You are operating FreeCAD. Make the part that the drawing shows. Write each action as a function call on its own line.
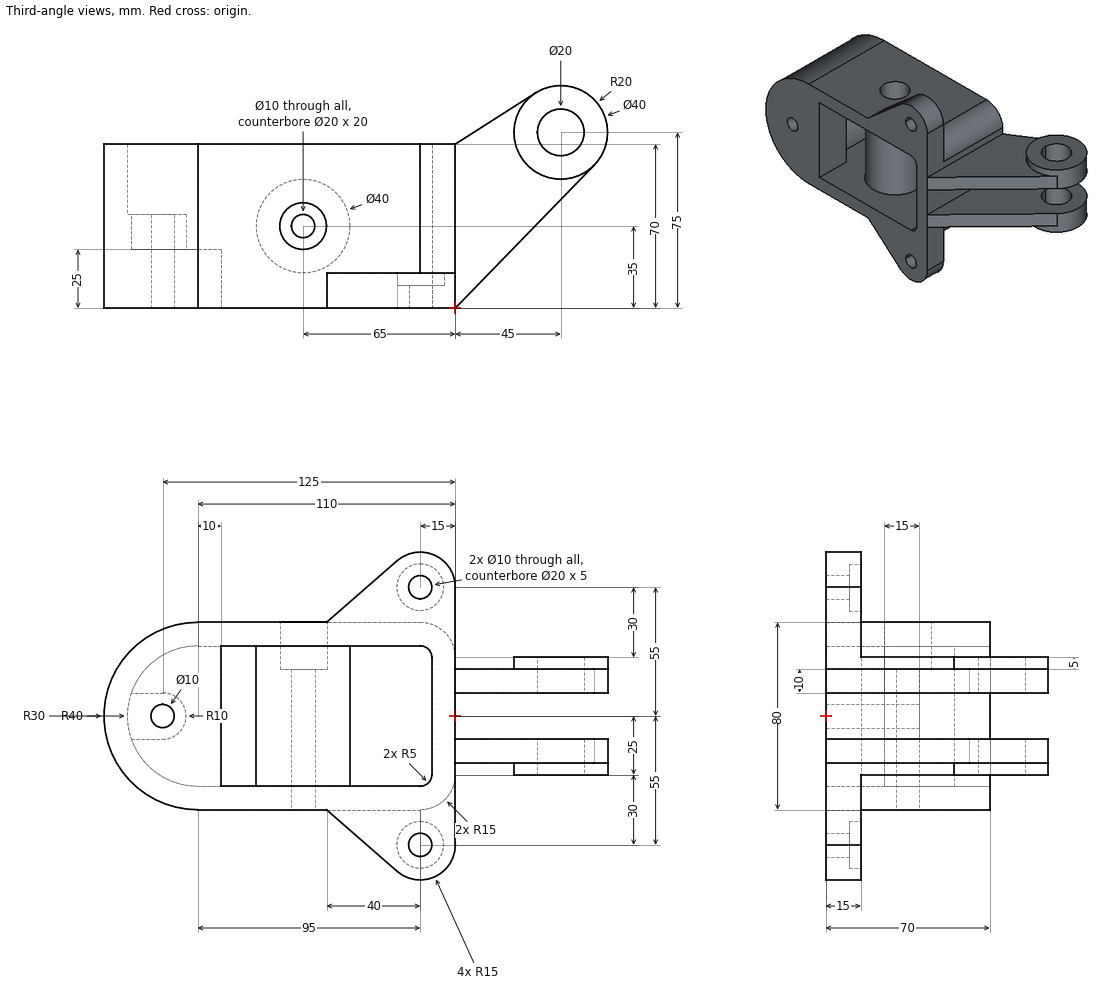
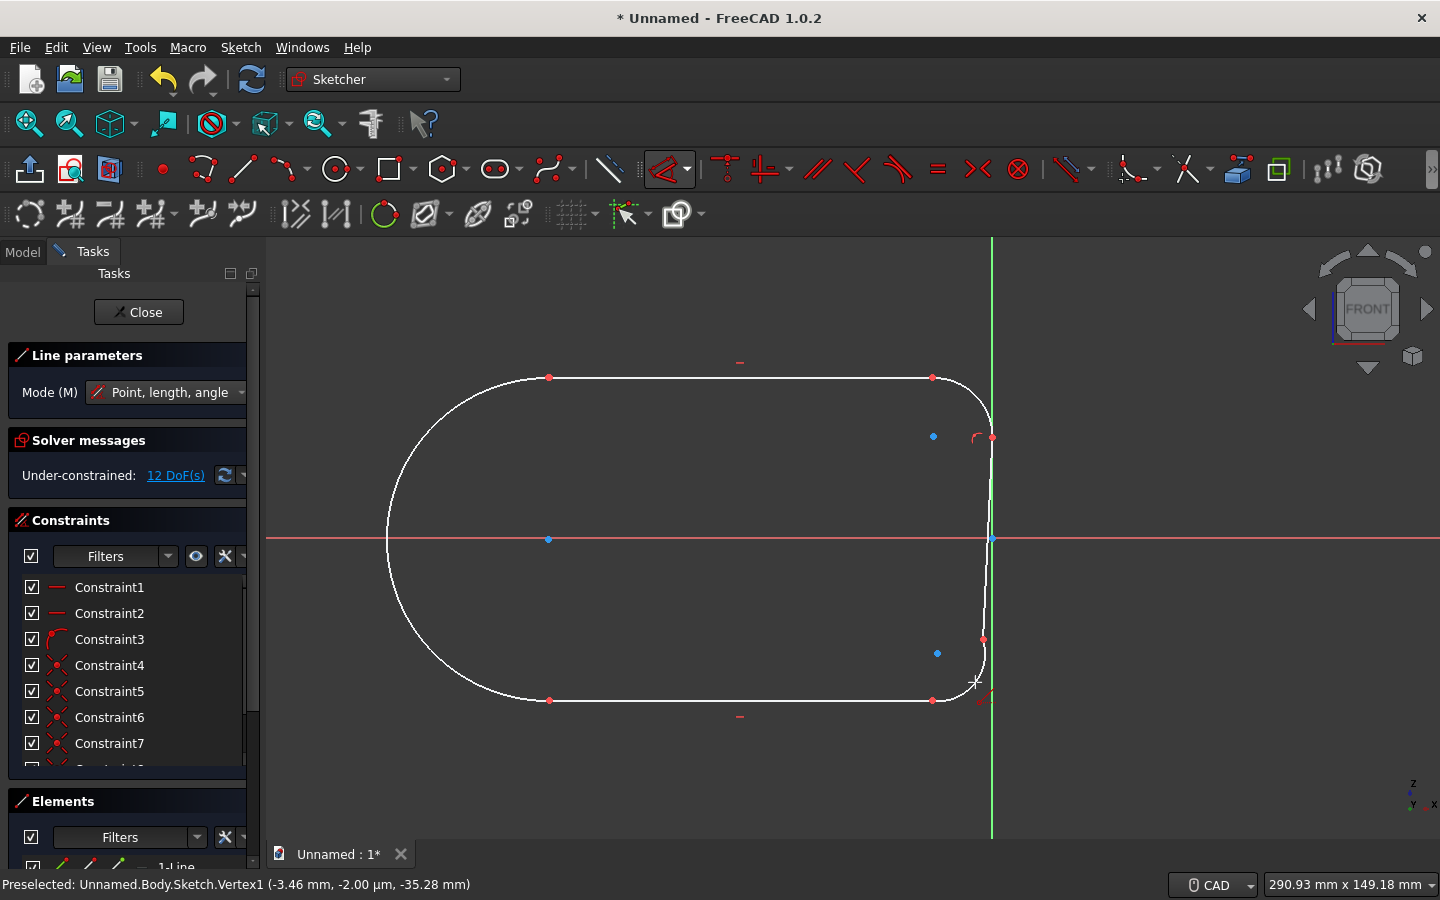
click(549, 659)
click(932, 659)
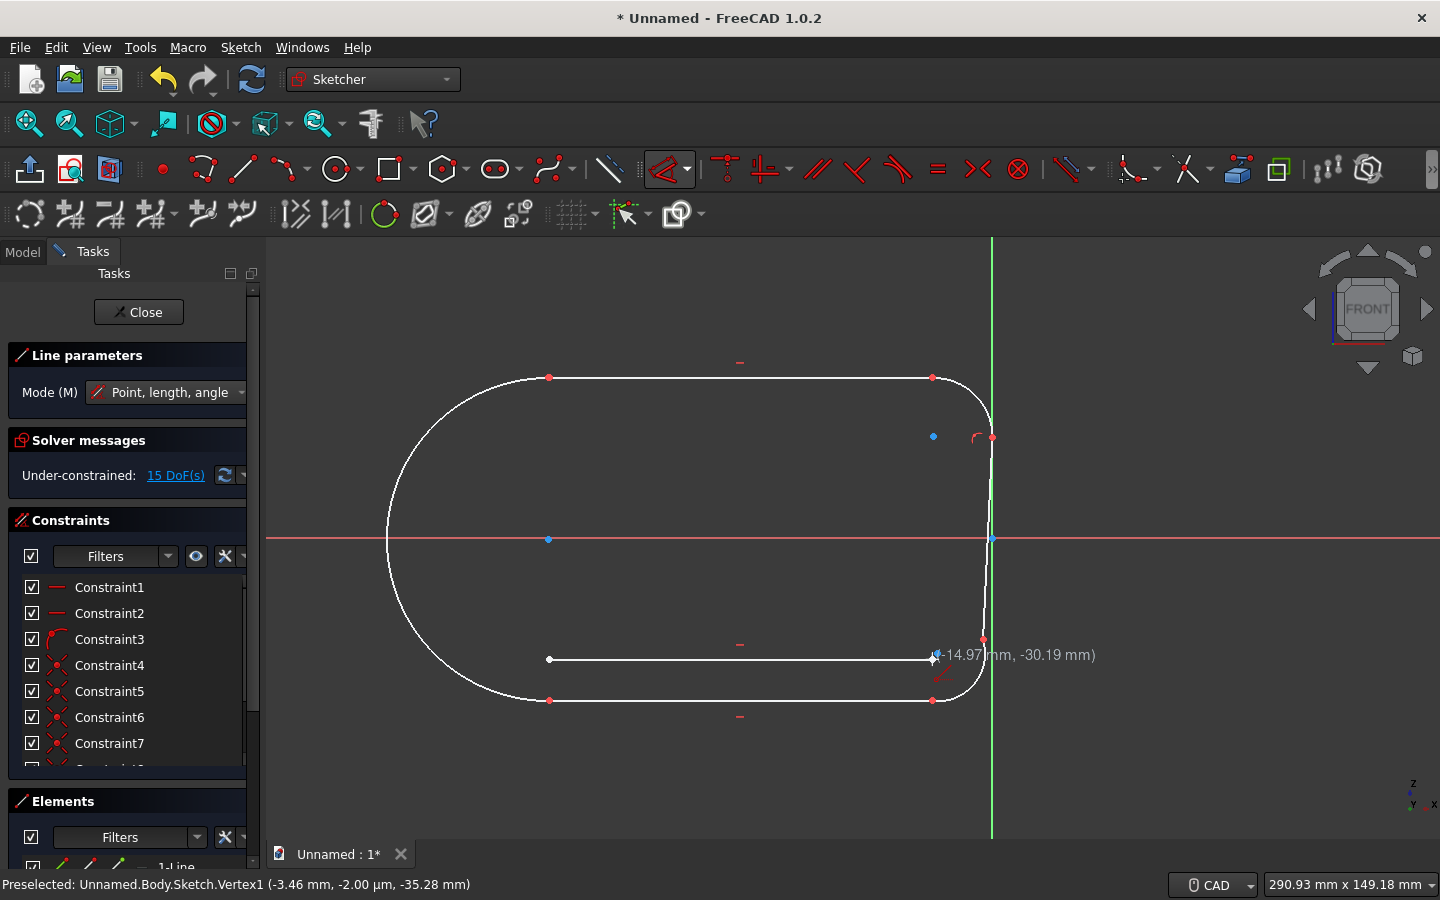
click(952, 639)
click(952, 437)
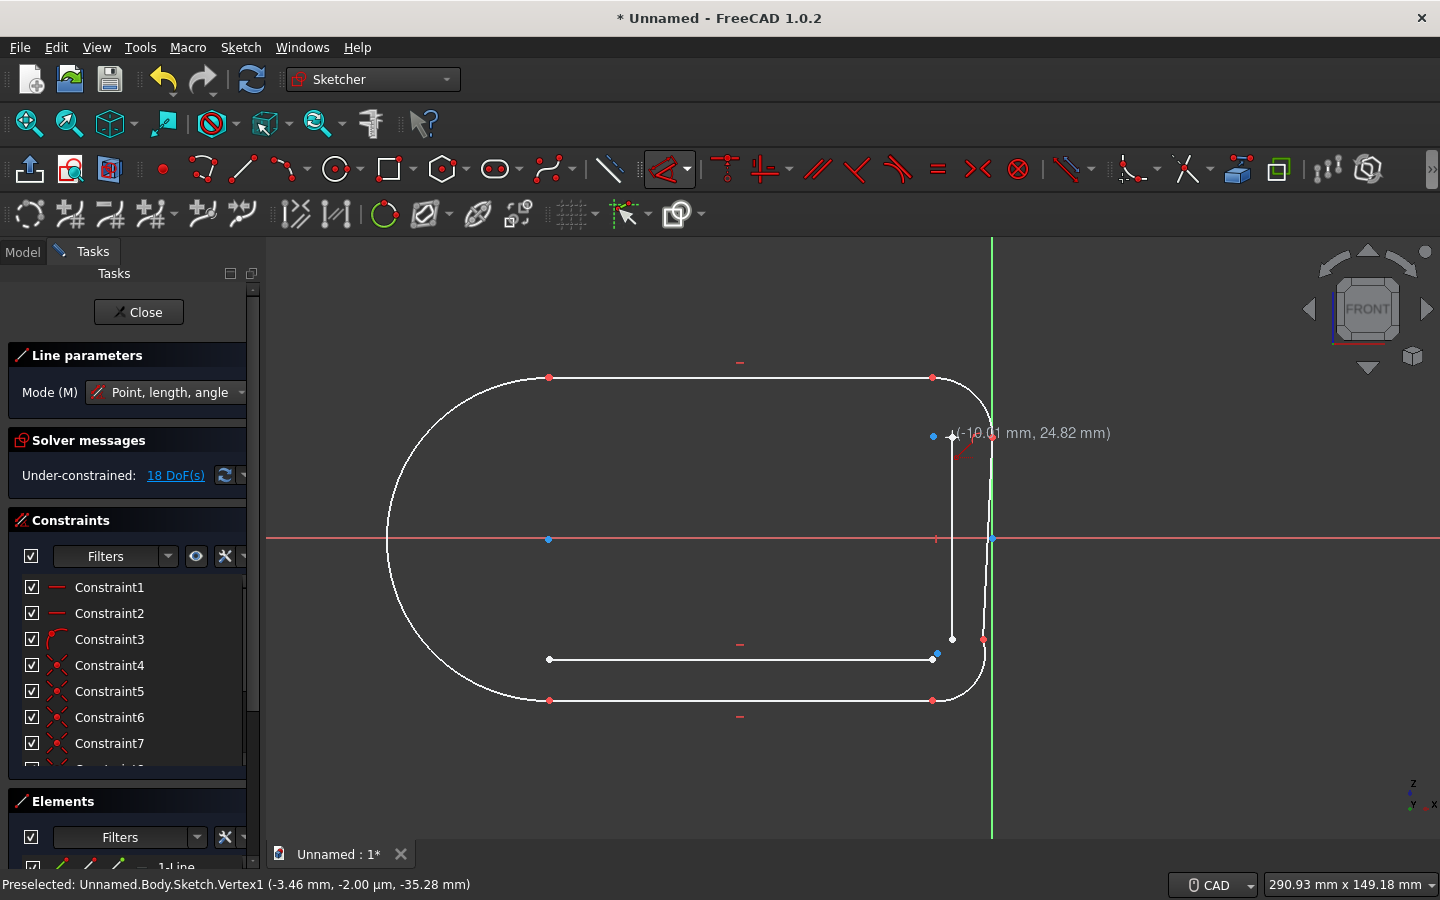
click(932, 417)
click(549, 417)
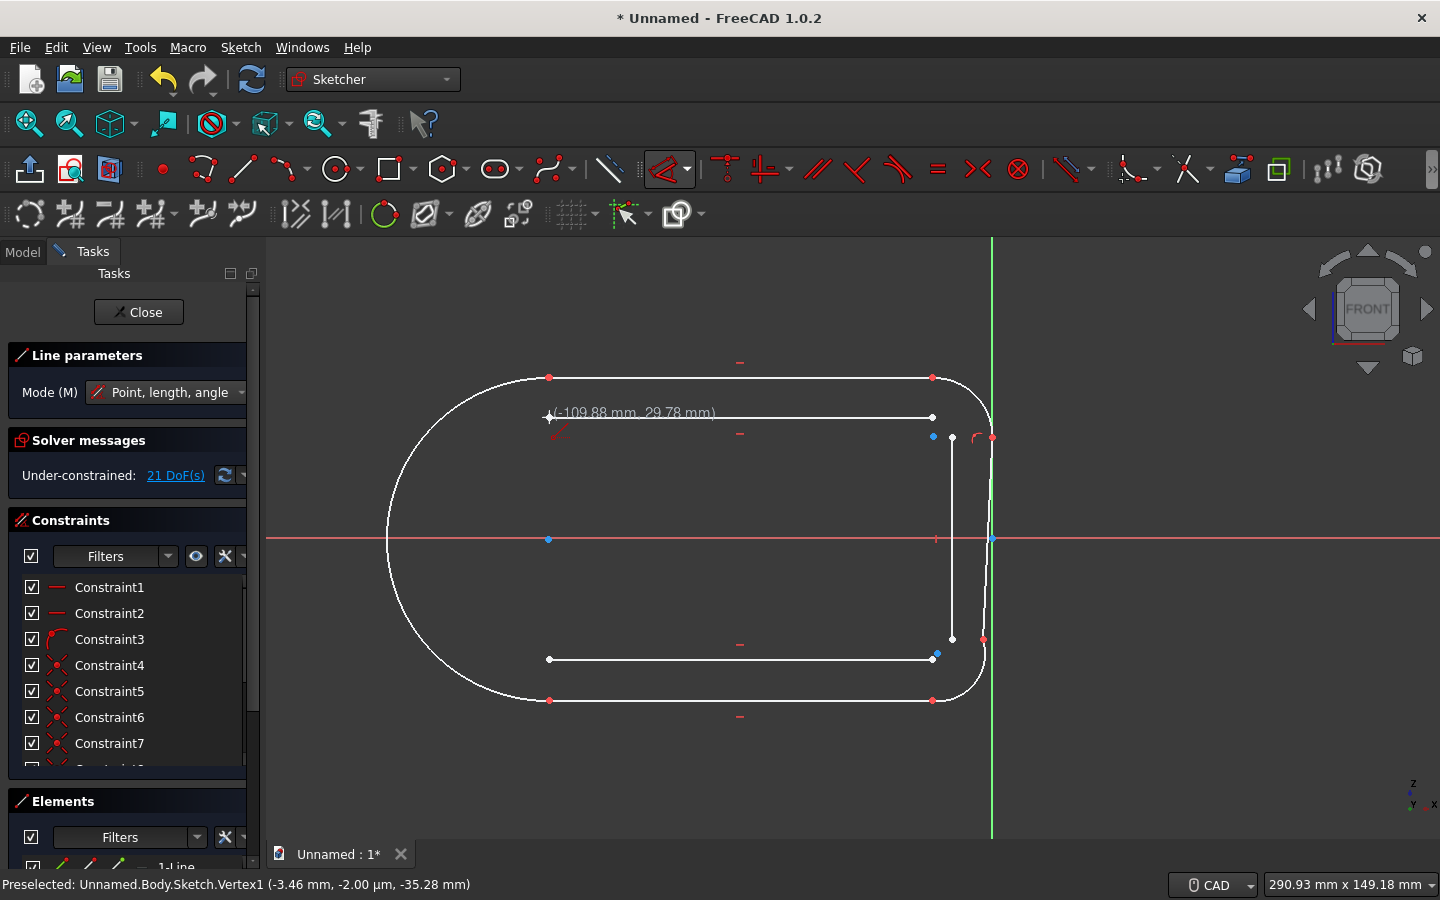
click(284, 170)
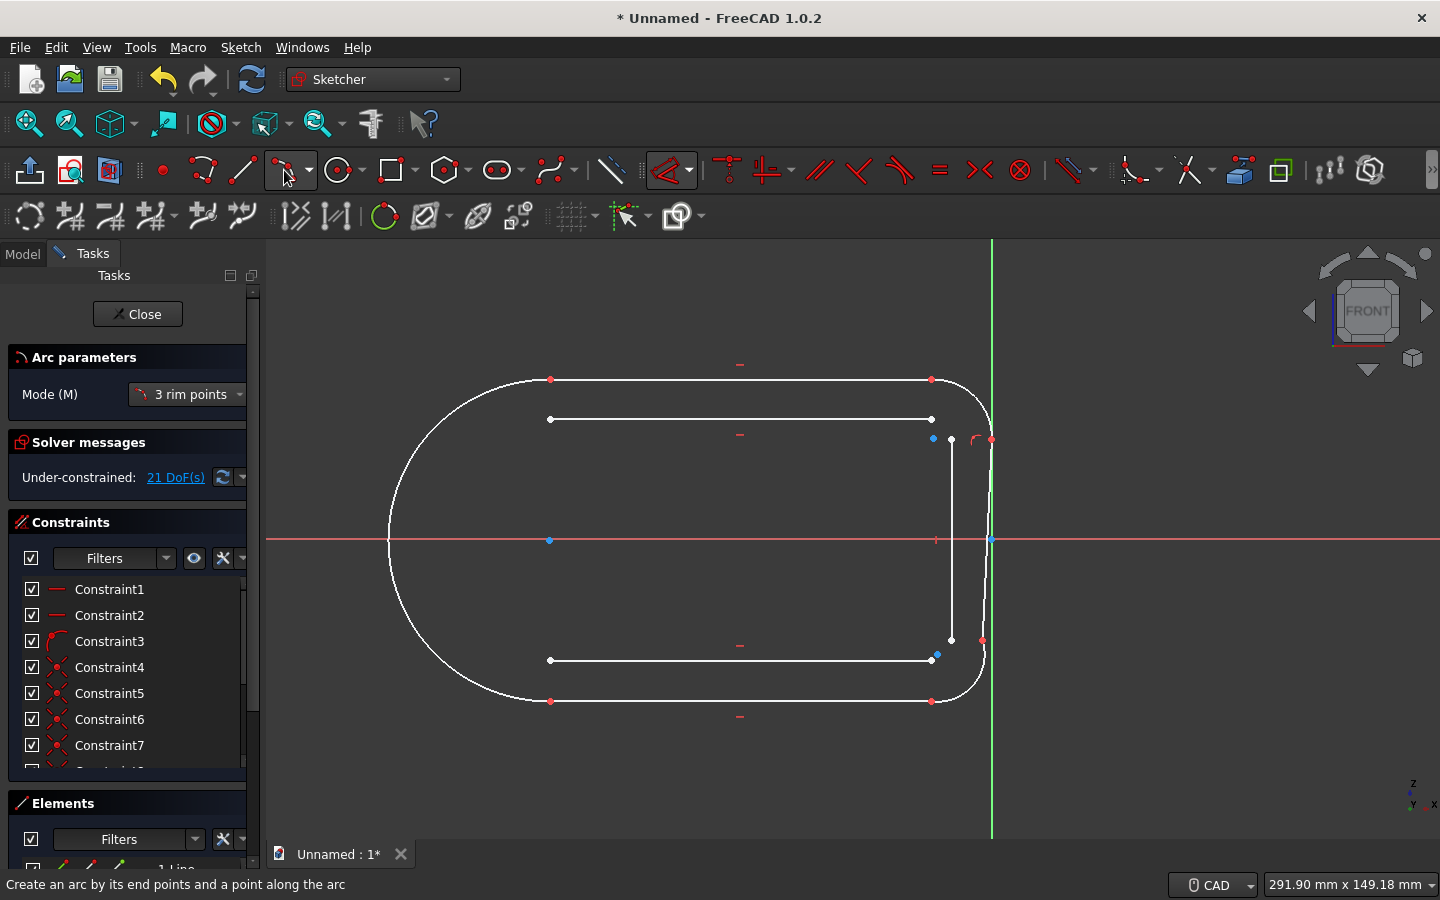
click(932, 661)
click(952, 641)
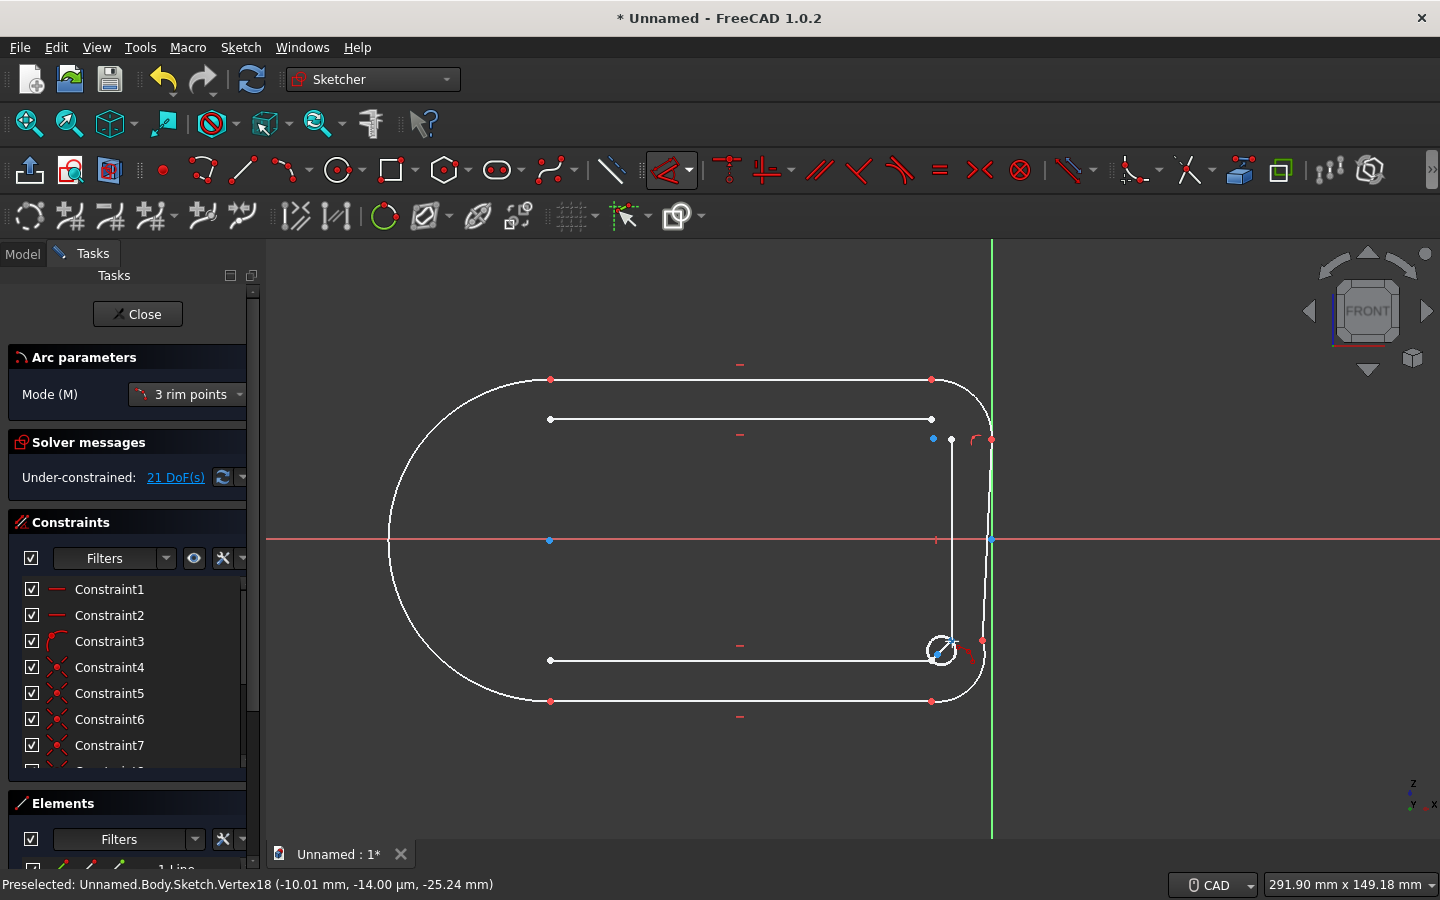
scroll(946, 654, up, 5)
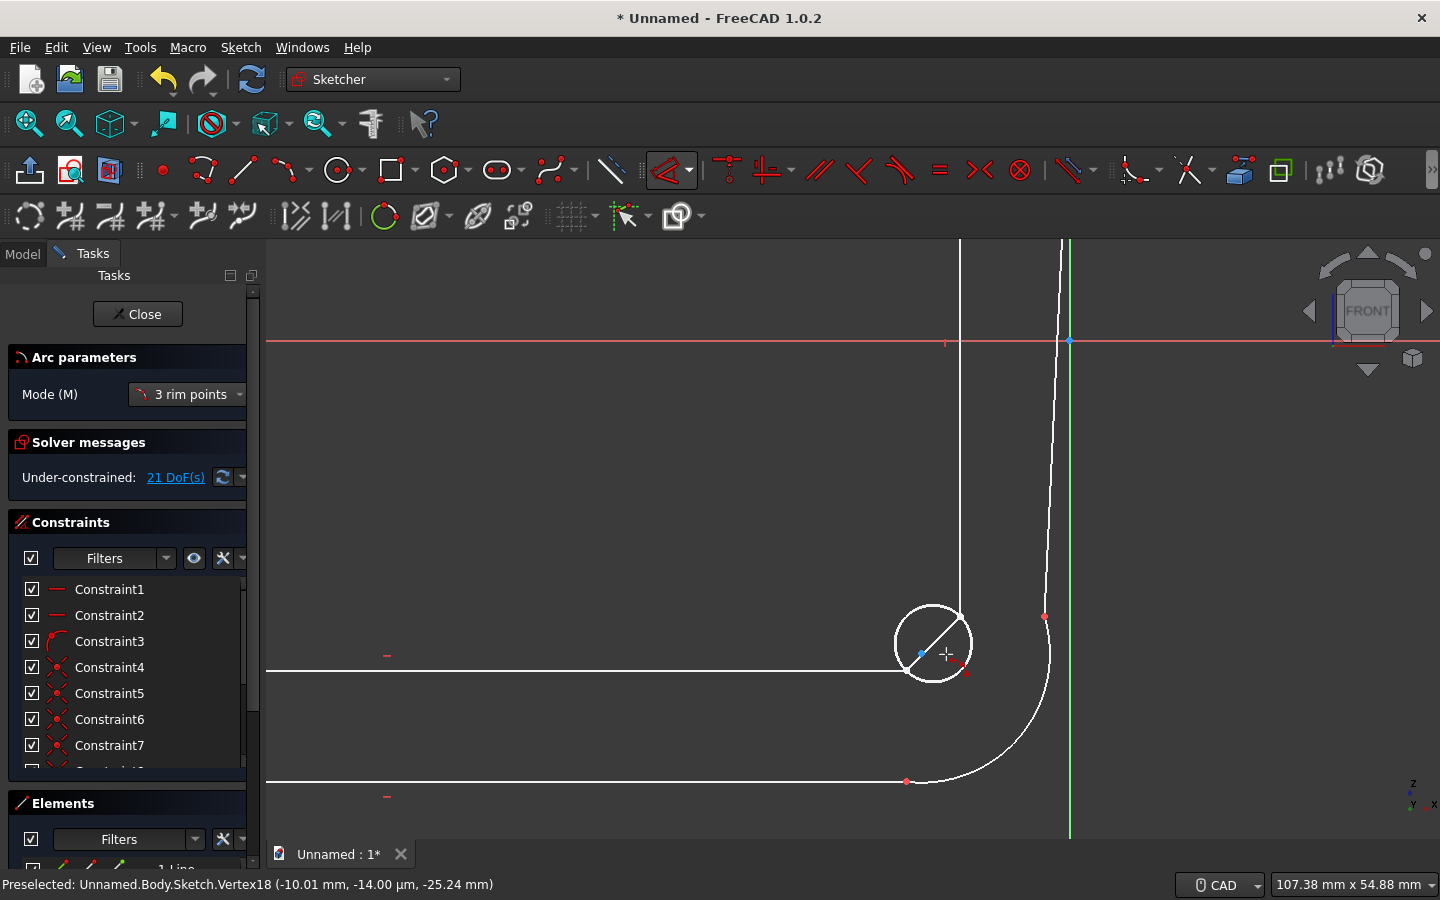
click(945, 653)